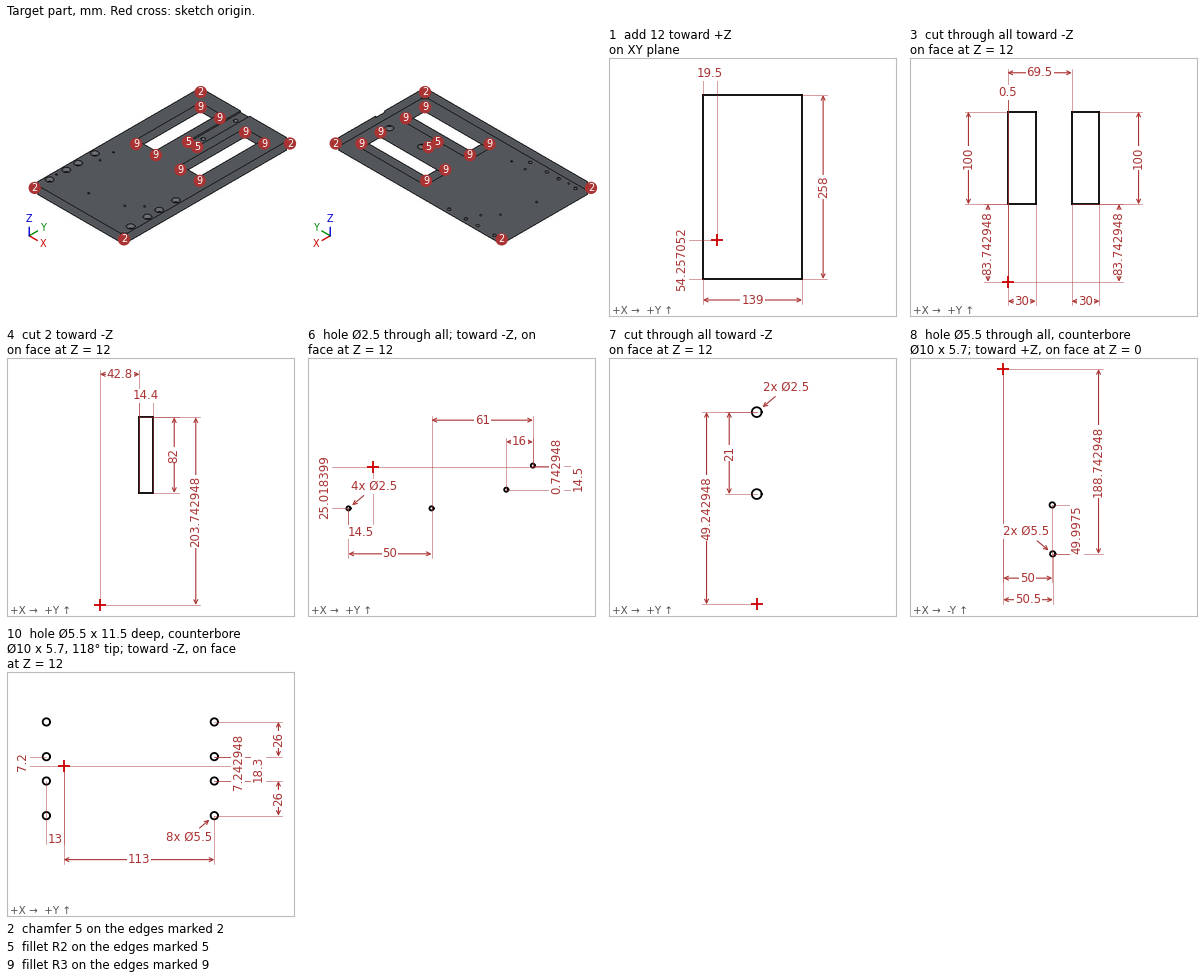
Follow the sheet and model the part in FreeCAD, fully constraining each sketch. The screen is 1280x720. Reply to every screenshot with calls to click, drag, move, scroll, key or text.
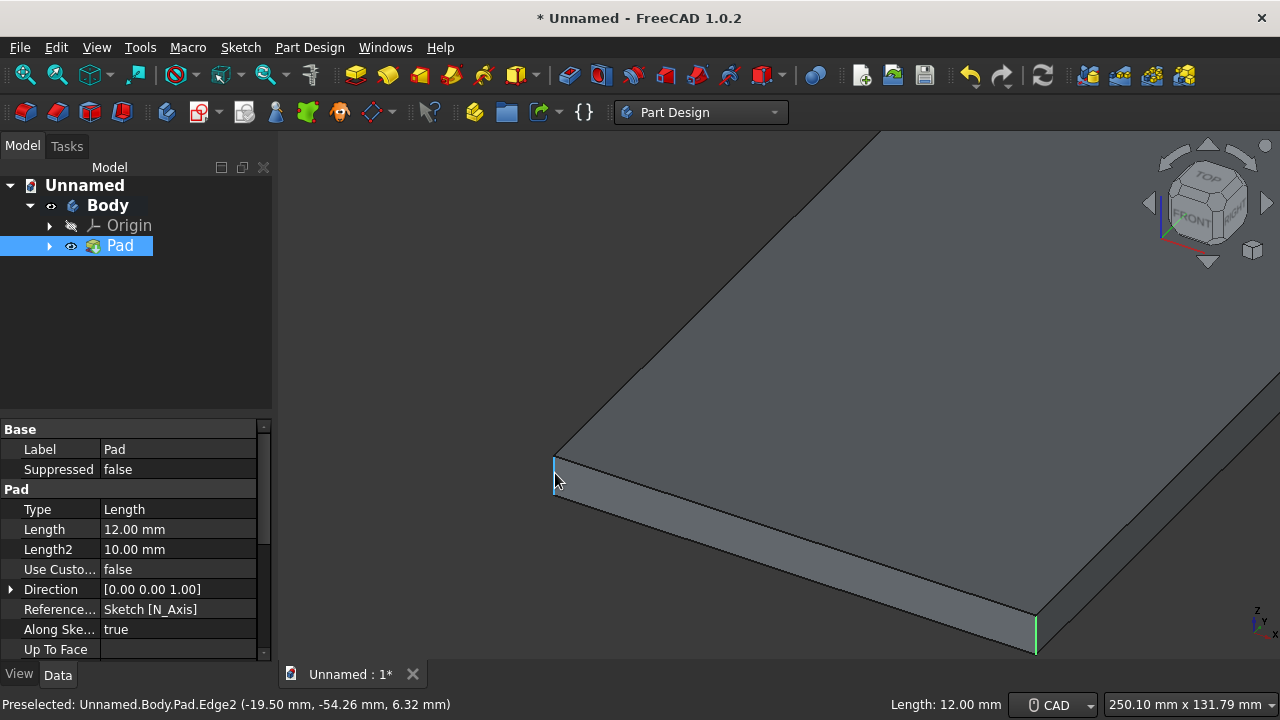
key(v)
key(f)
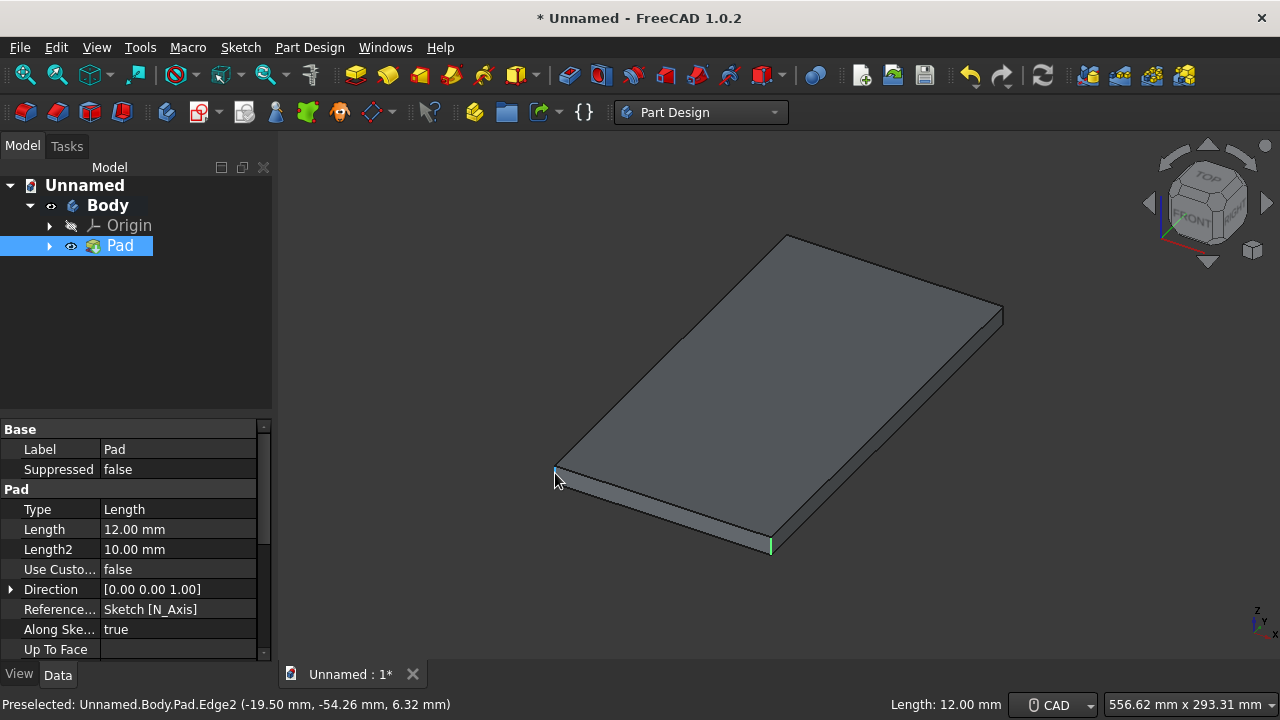
key(0)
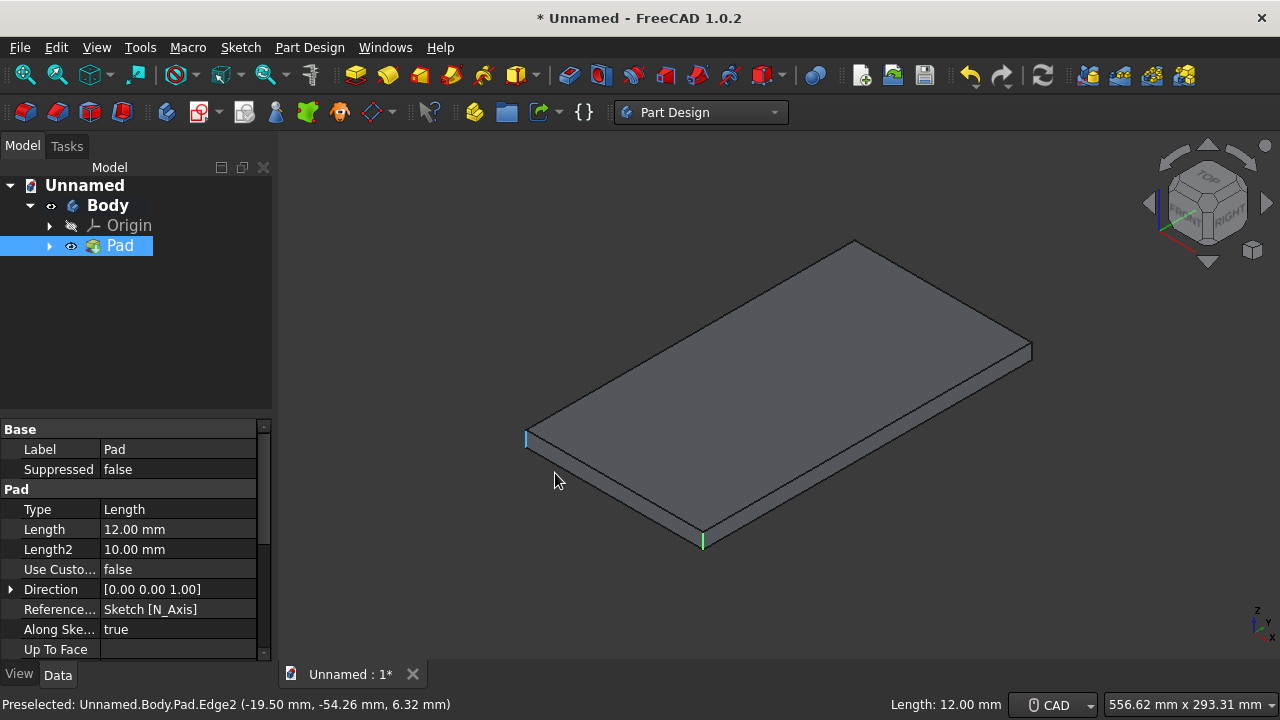
scroll(526, 438, up, 4)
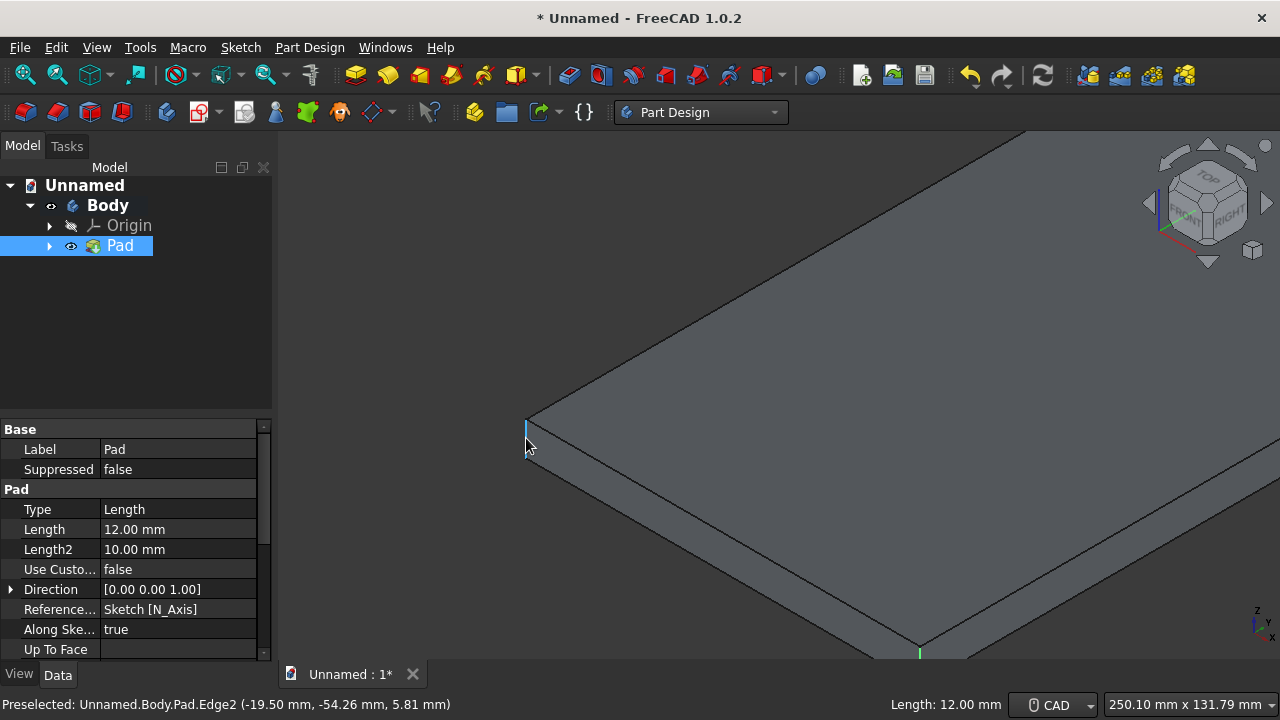
key(v)
key(f)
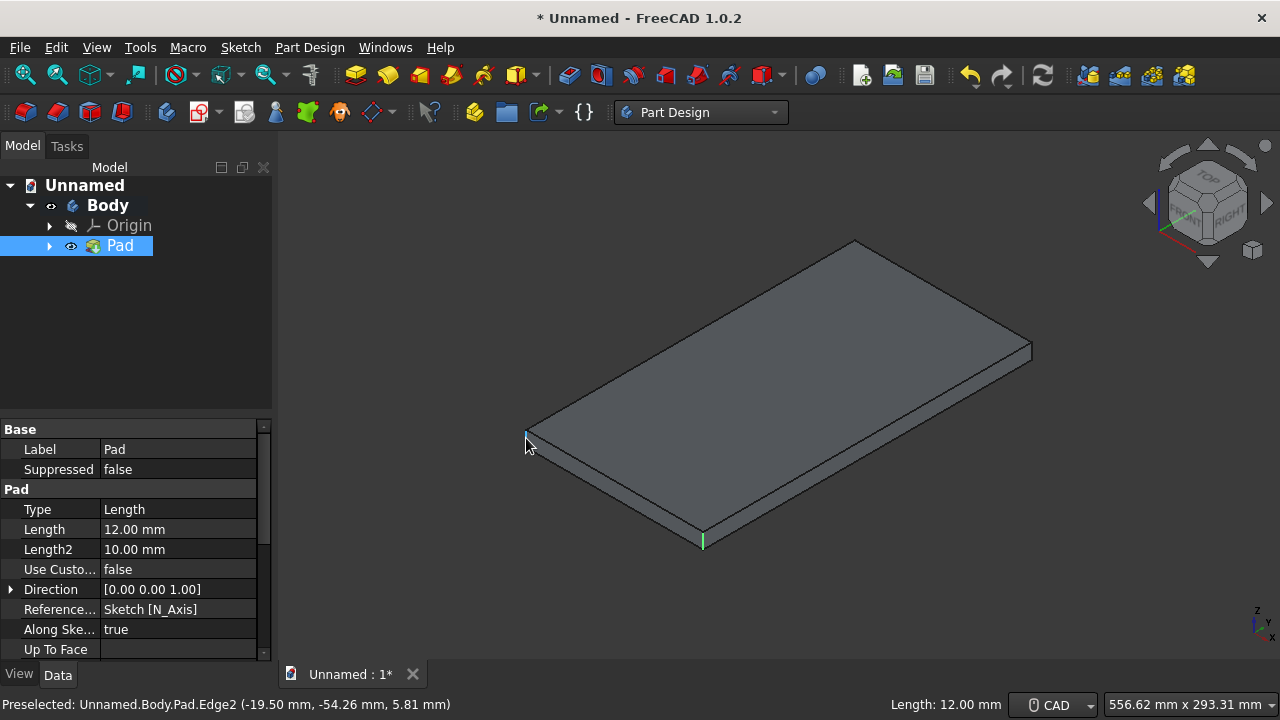
key(2)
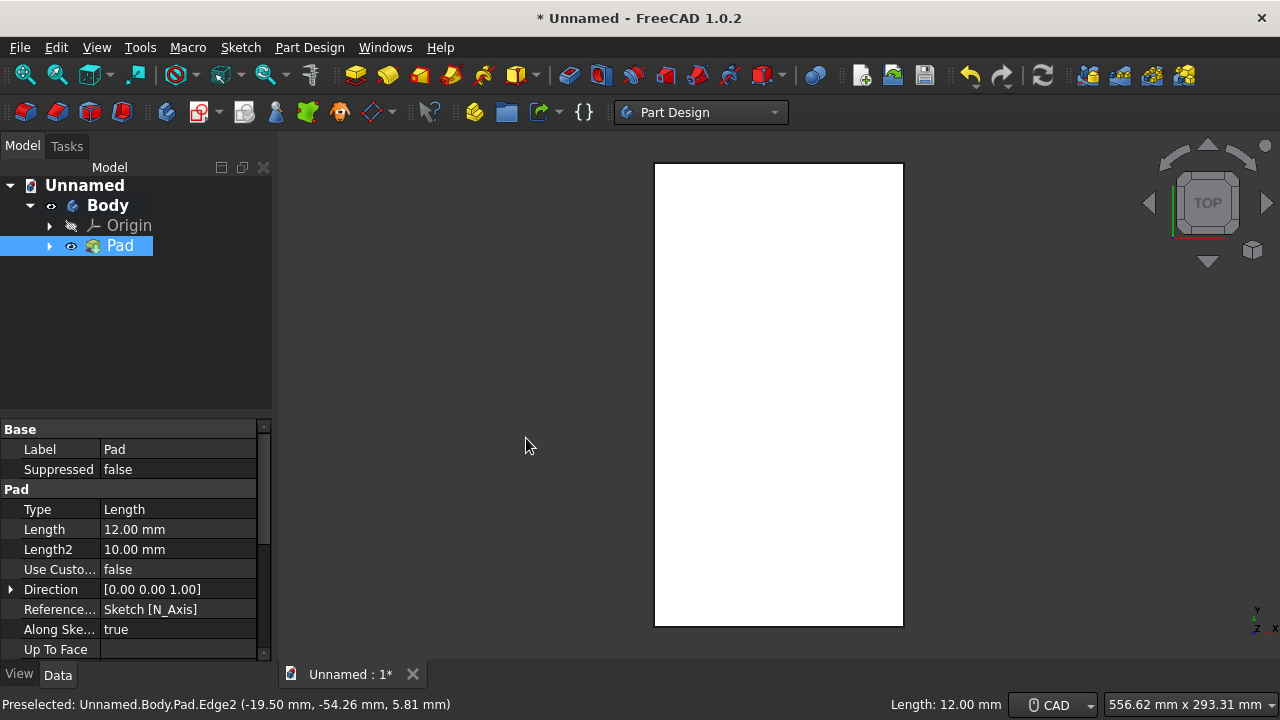
scroll(654, 626, up, 4)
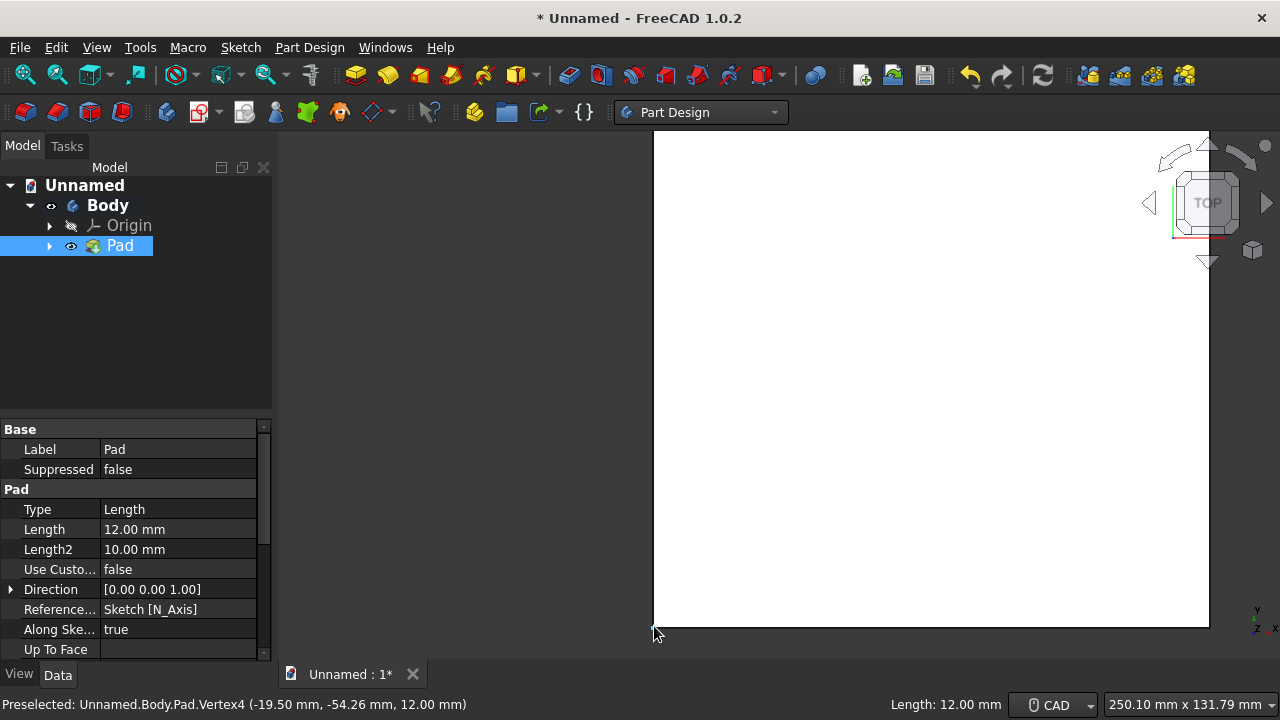
key(v)
key(f)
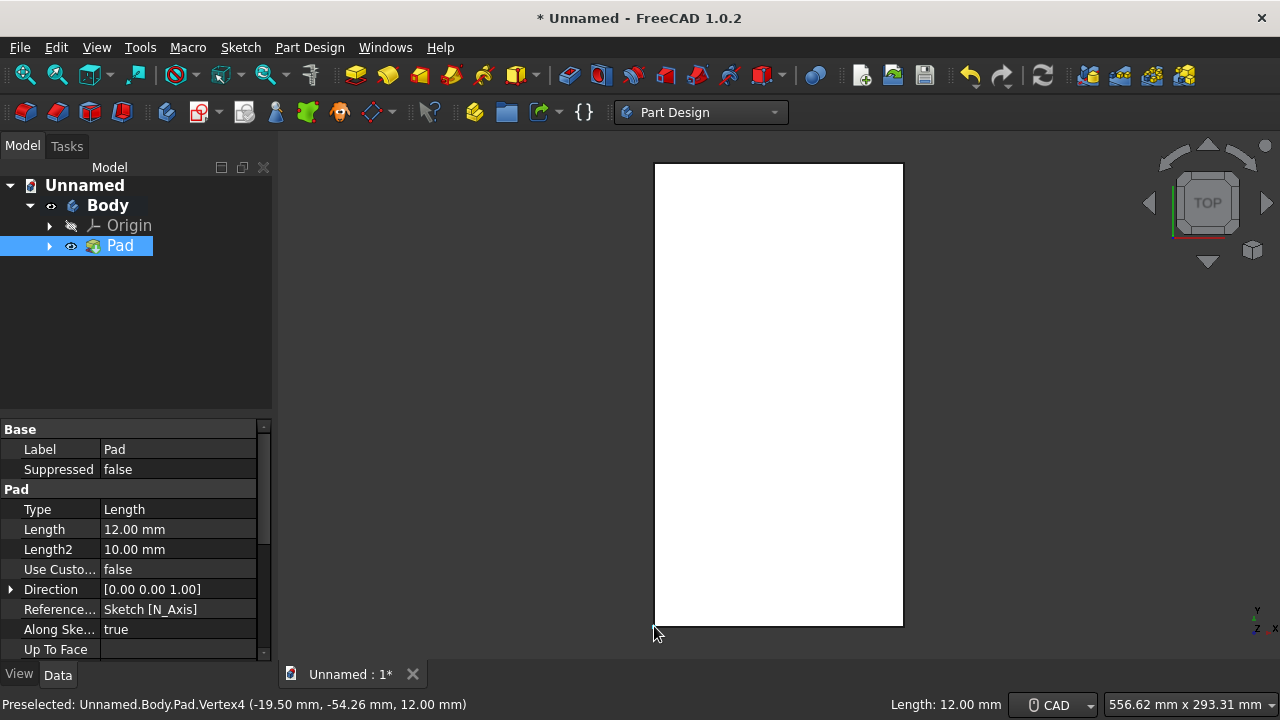
key(1)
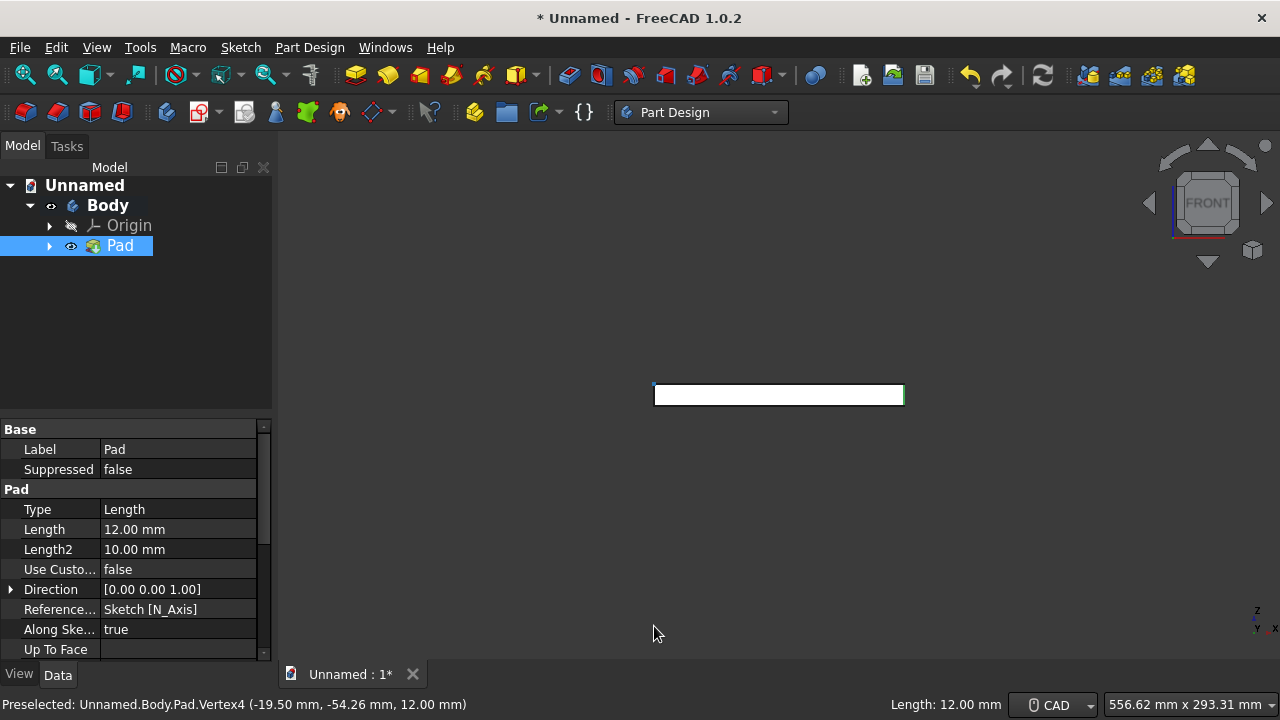
click(26, 76)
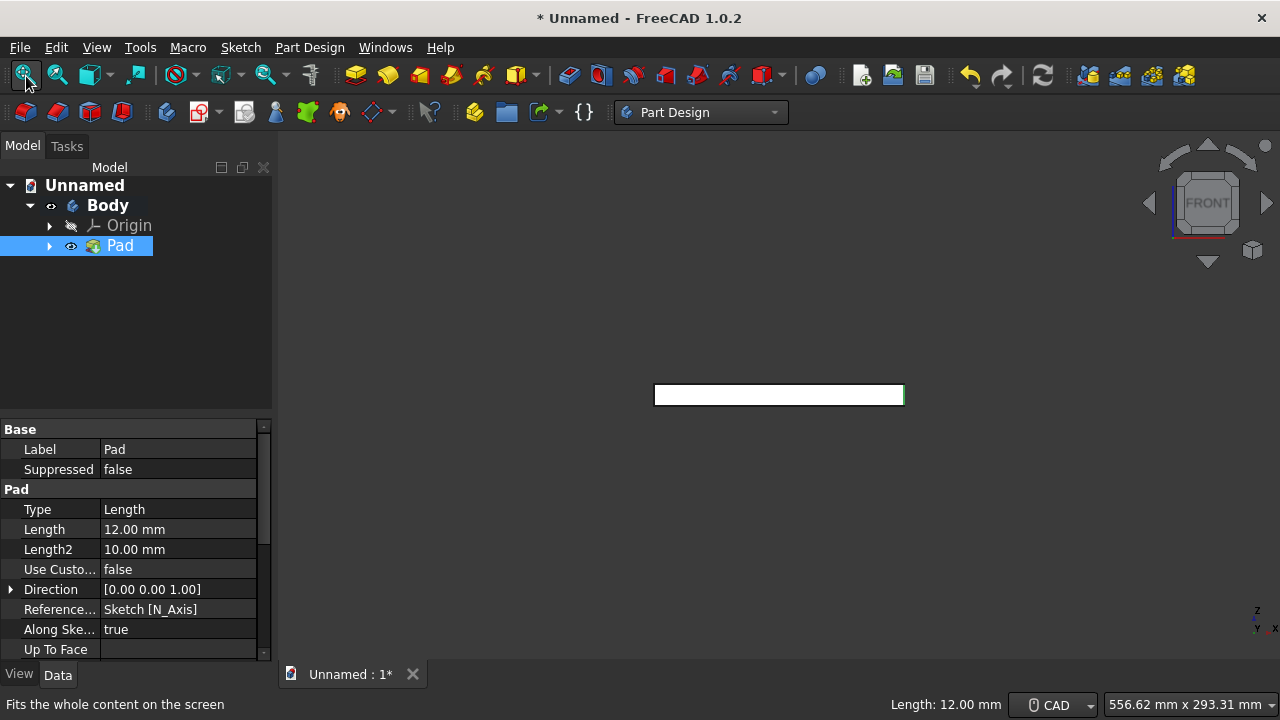
click(654, 394, ctrl)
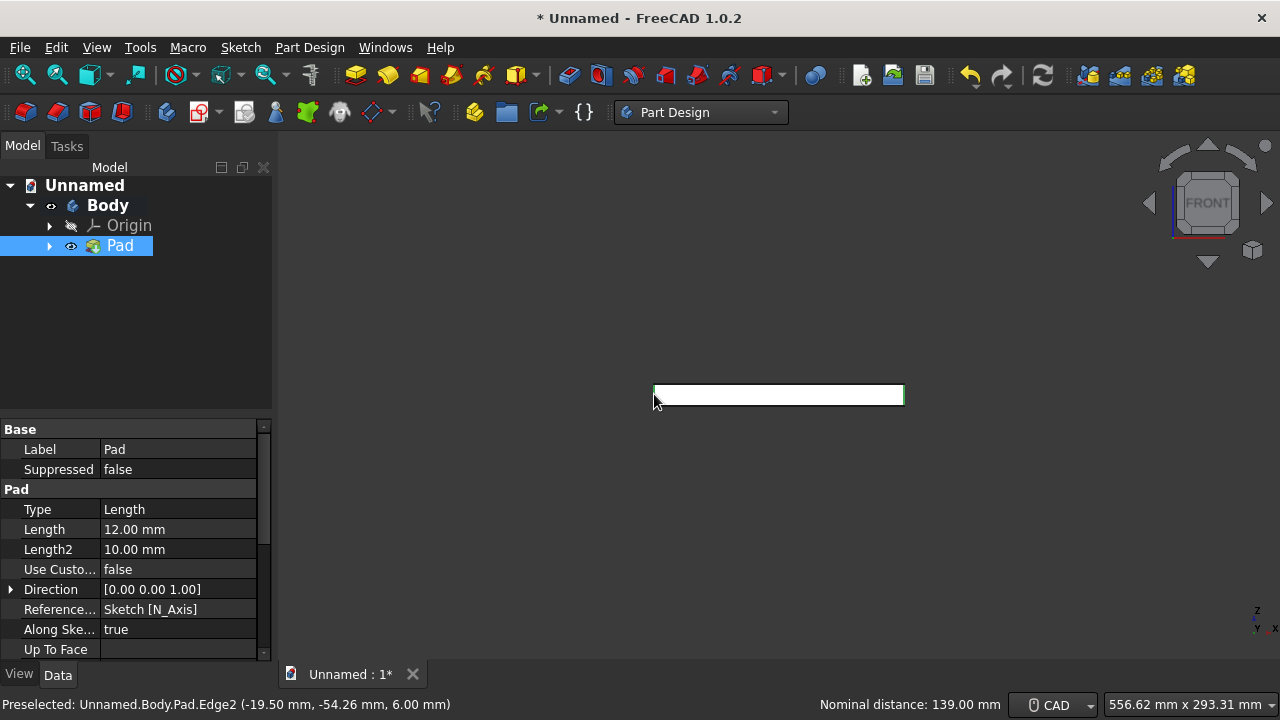
scroll(654, 394, up, 4)